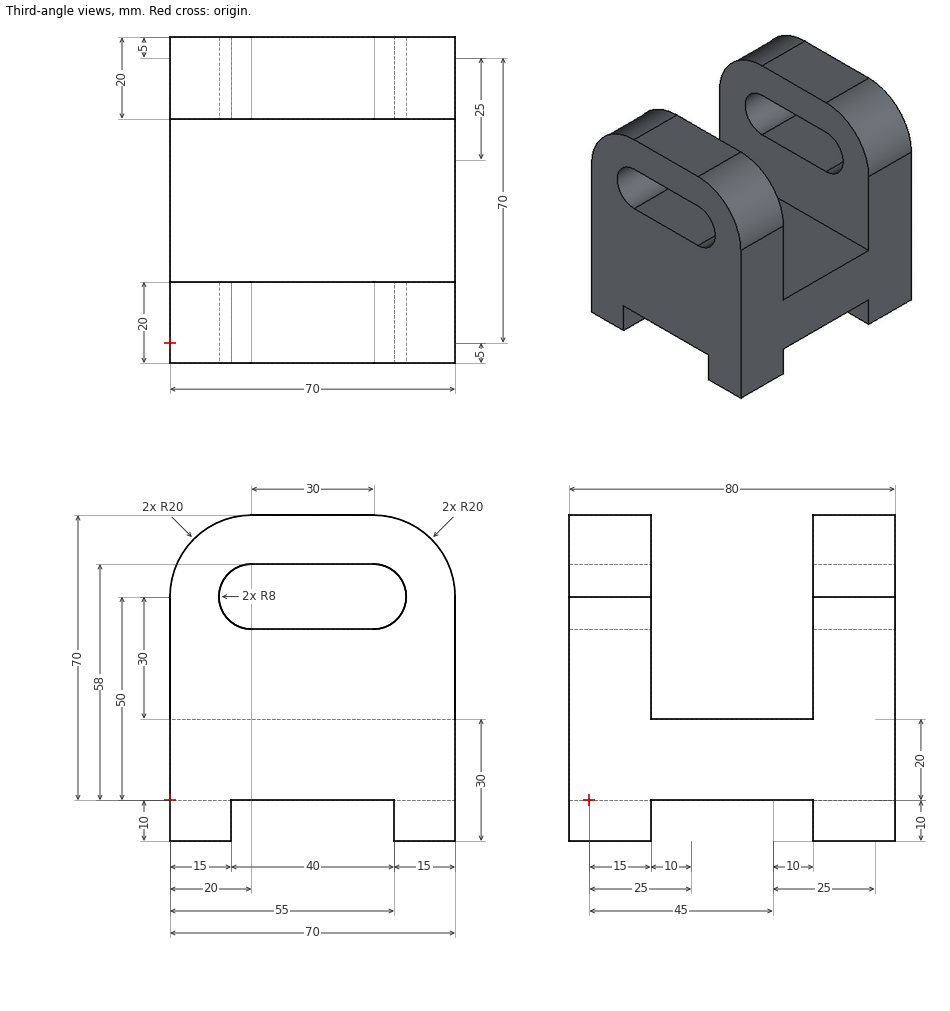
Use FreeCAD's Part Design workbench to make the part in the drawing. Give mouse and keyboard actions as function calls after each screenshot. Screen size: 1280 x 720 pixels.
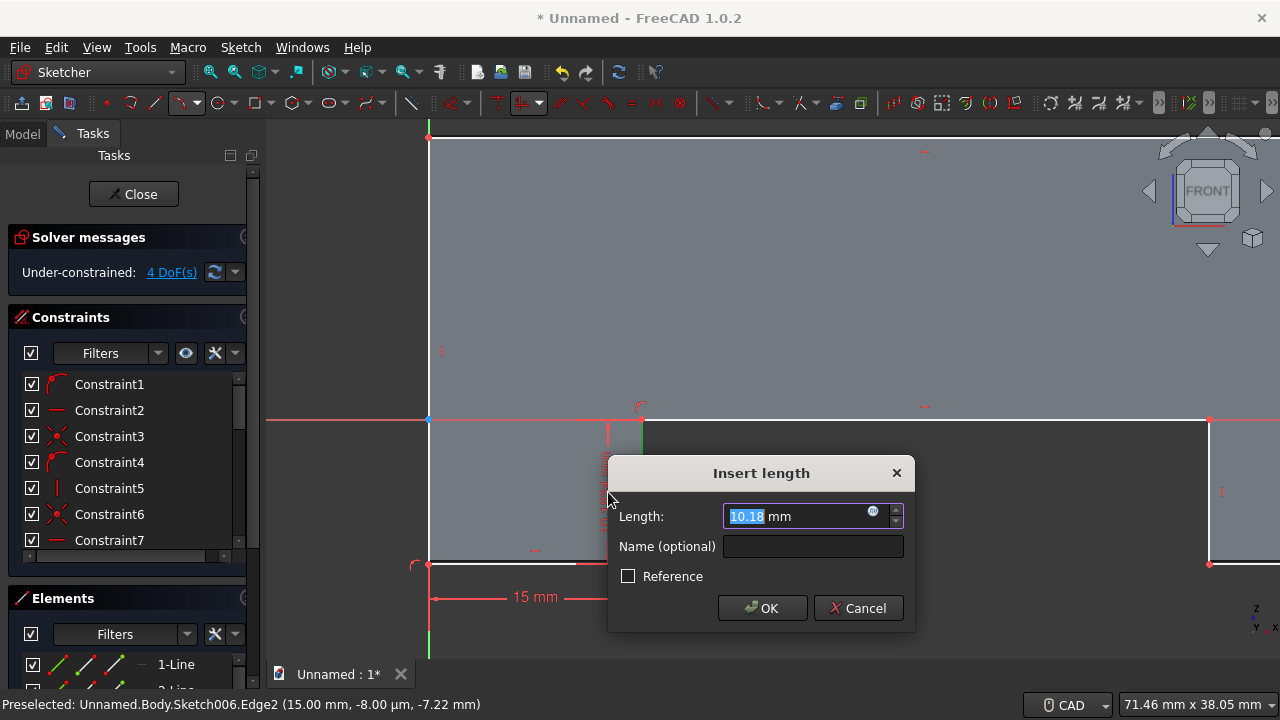
text(10)
key(Return)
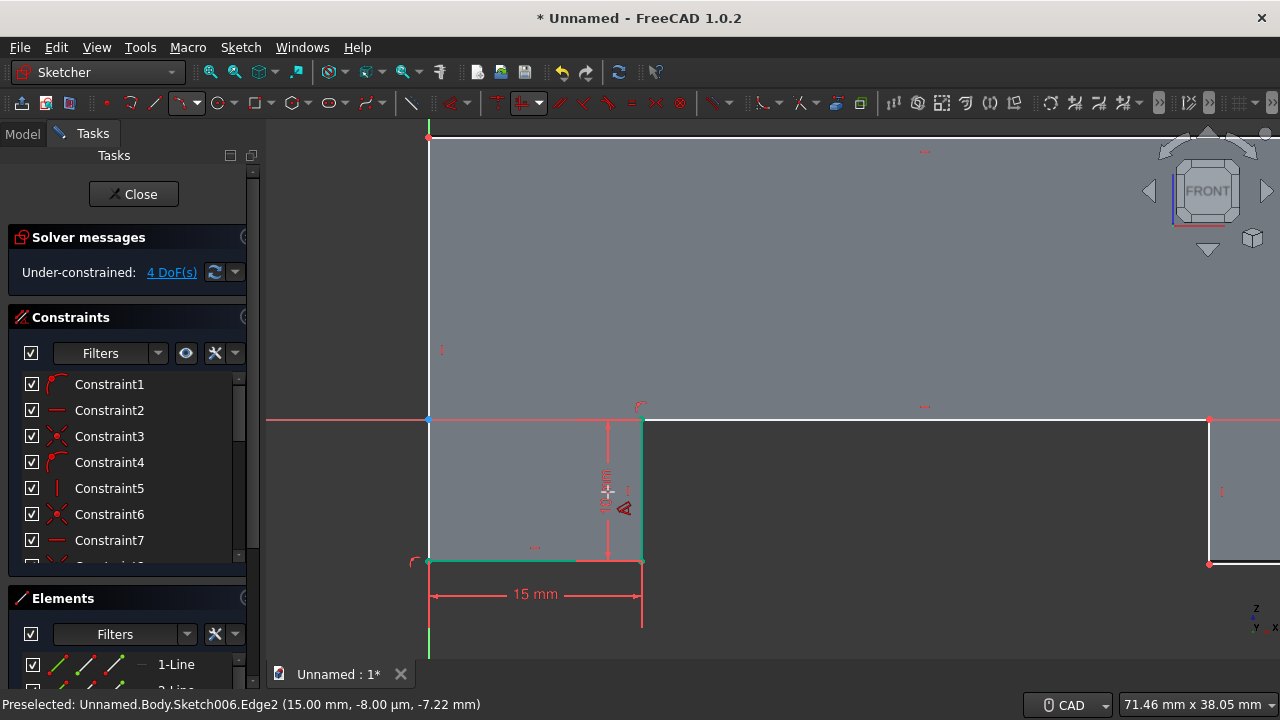
click(812, 420)
click(878, 454)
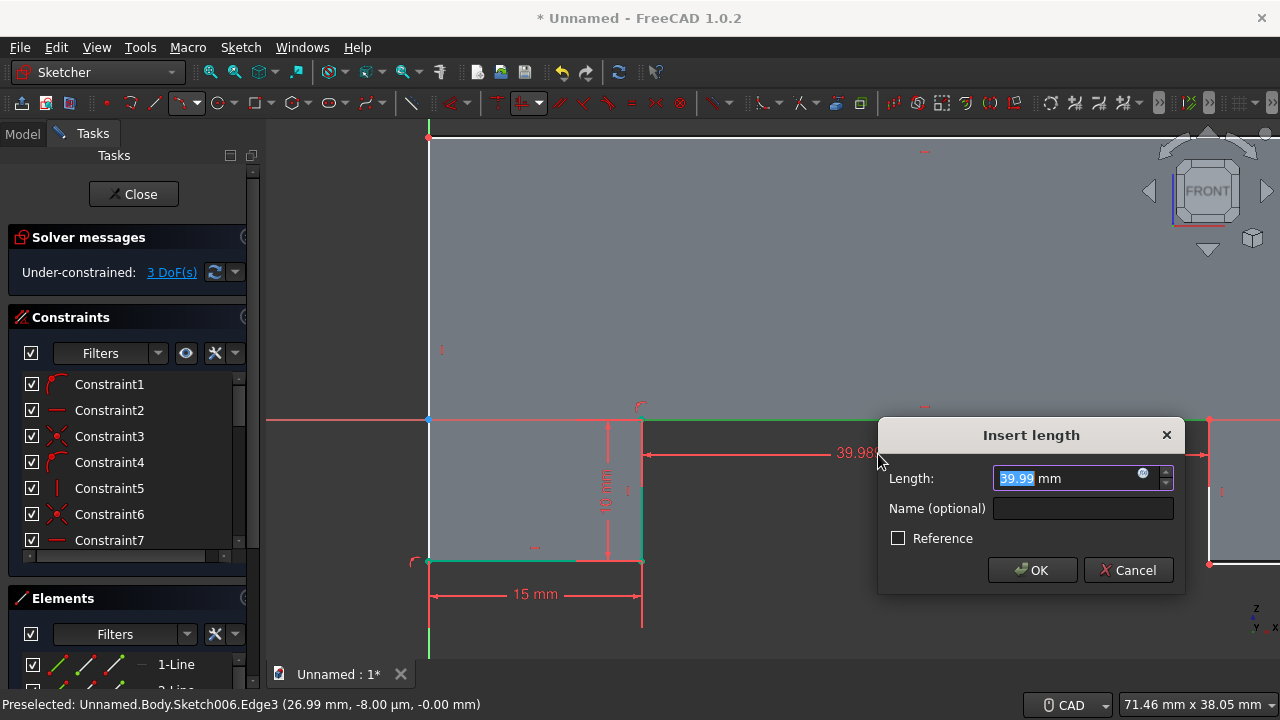
text(40)
key(Return)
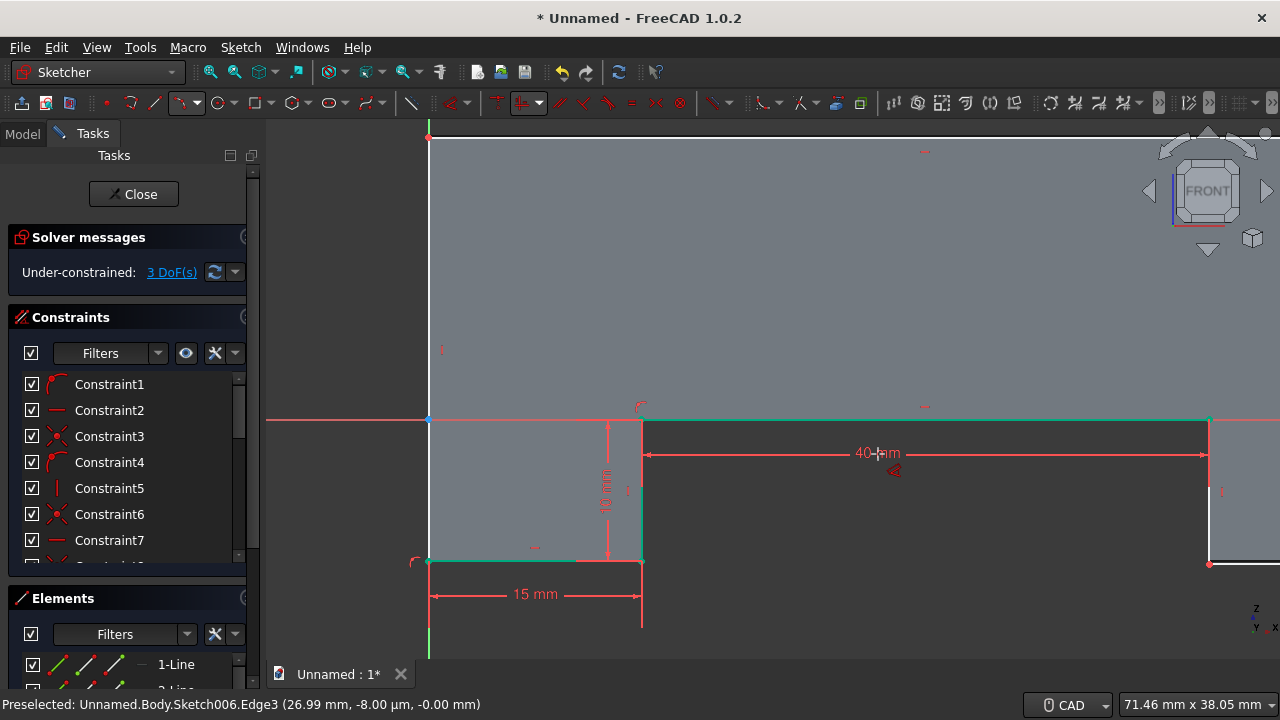
scroll(436, 438, down, 3)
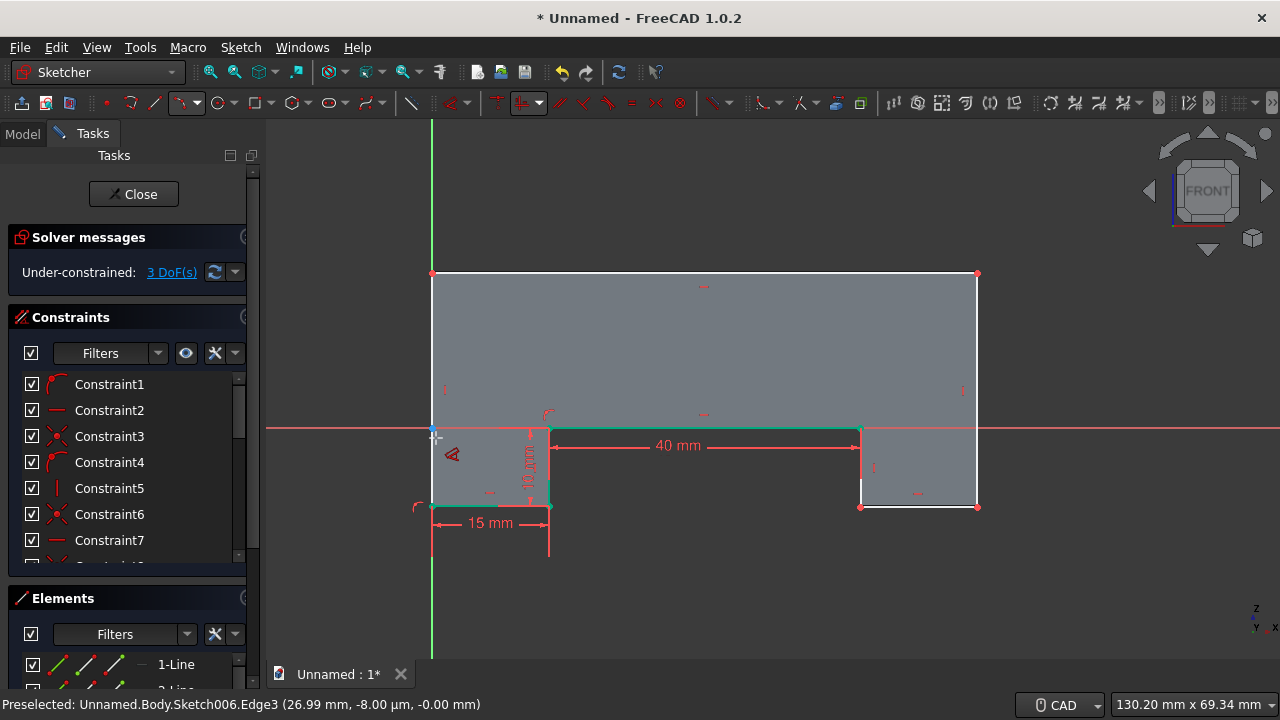
click(861, 452)
click(895, 468)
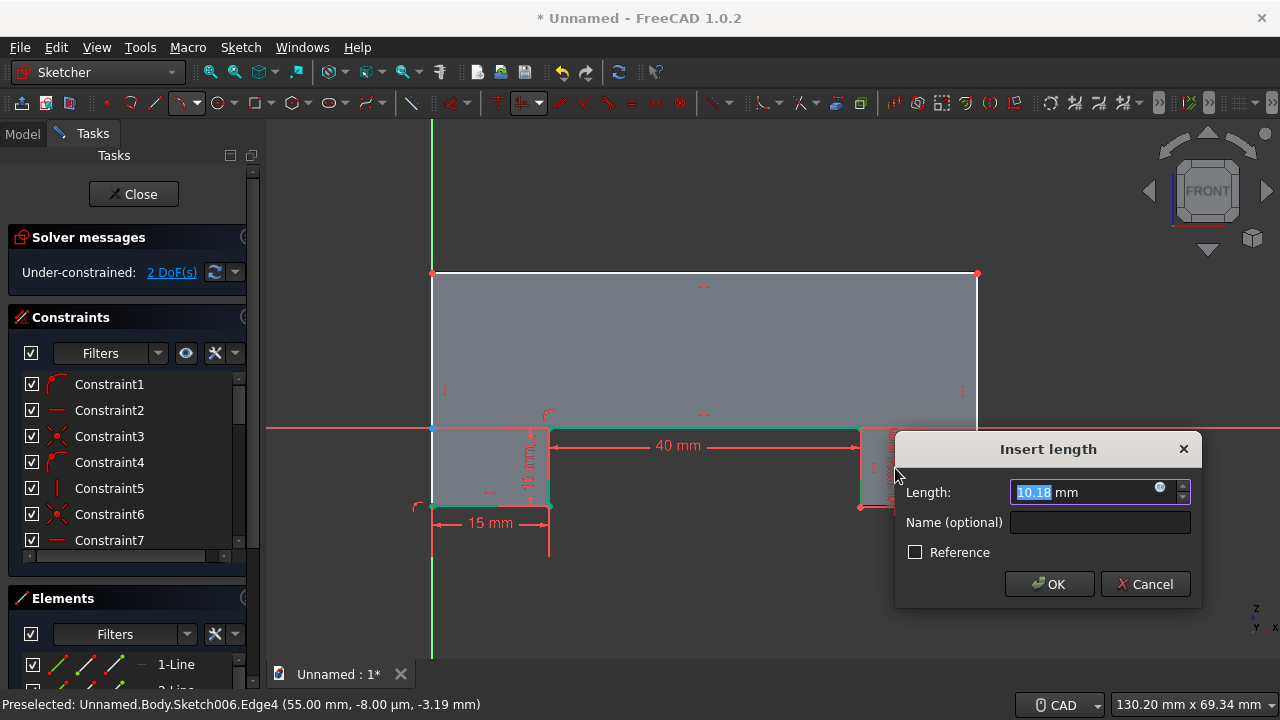
text(10)
key(Return)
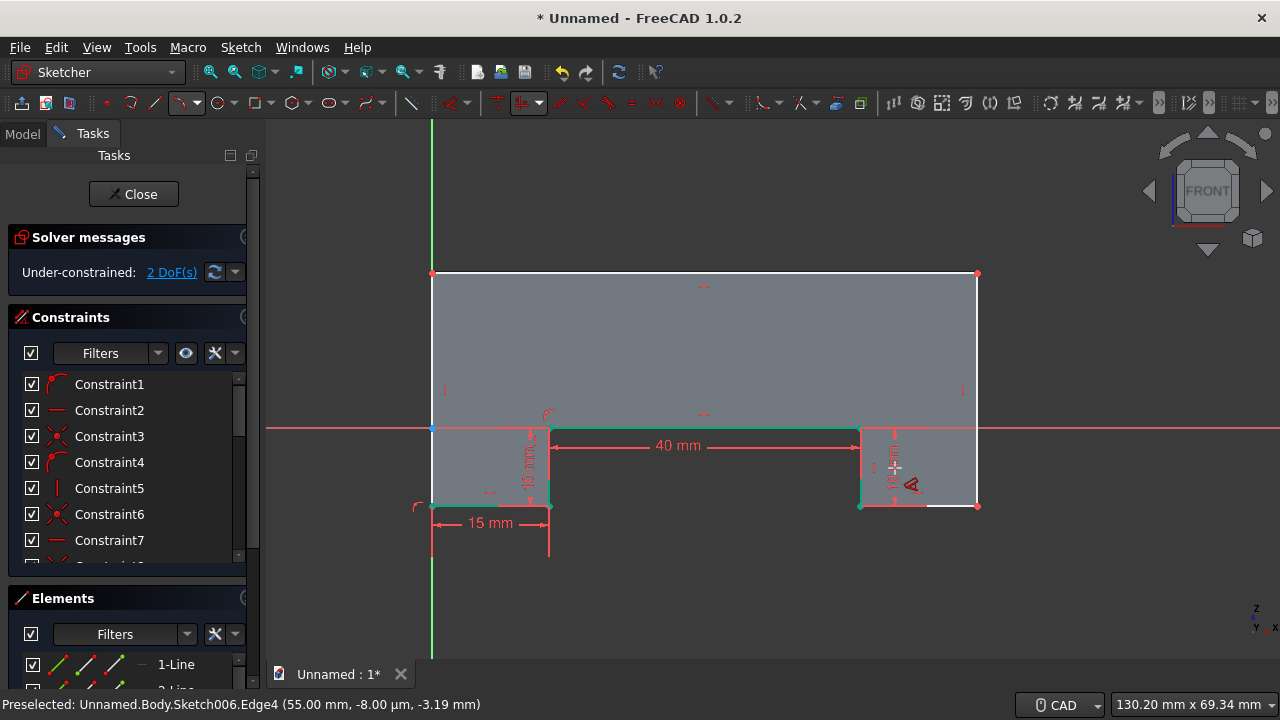
click(896, 506)
click(919, 540)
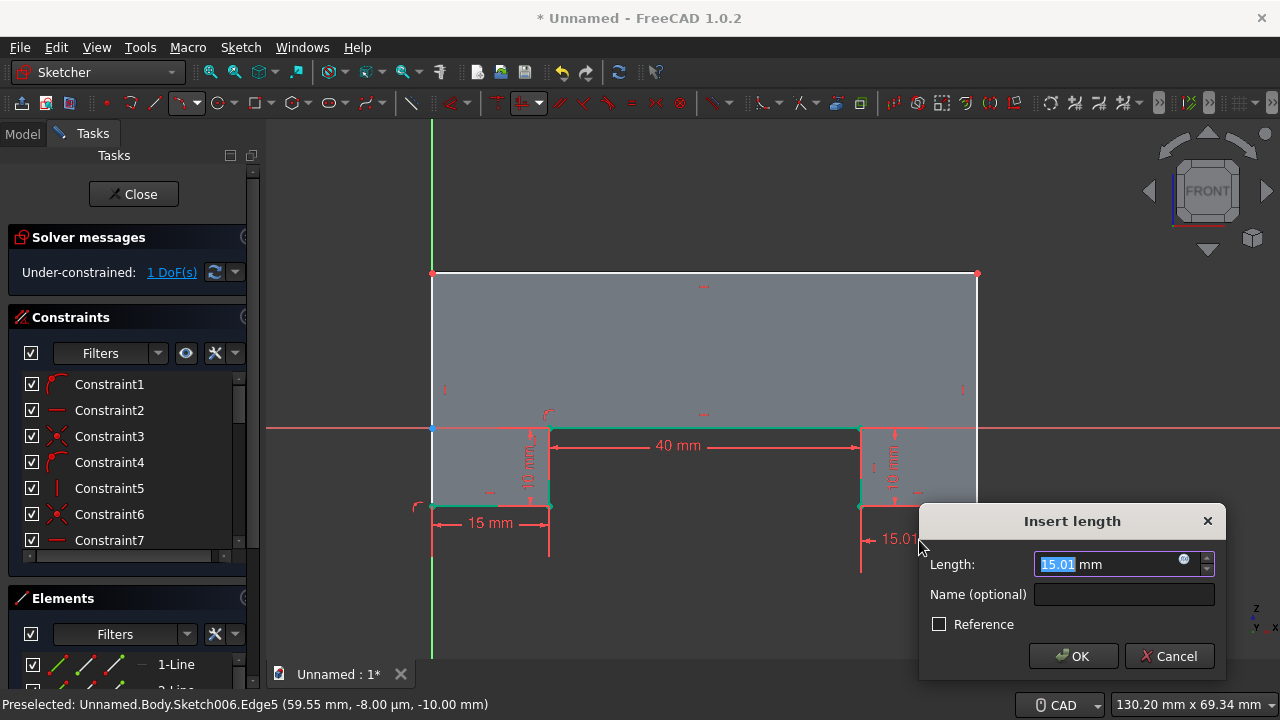
text(15)
key(Return)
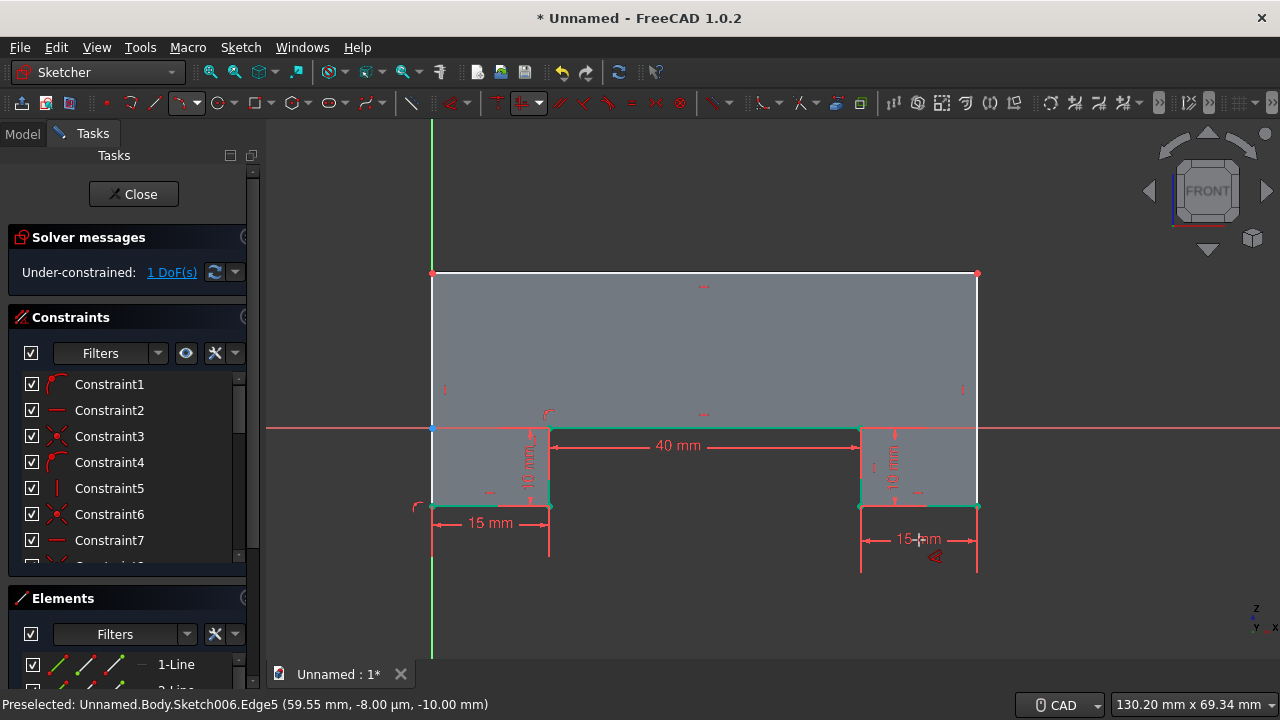
click(977, 343)
click(1011, 390)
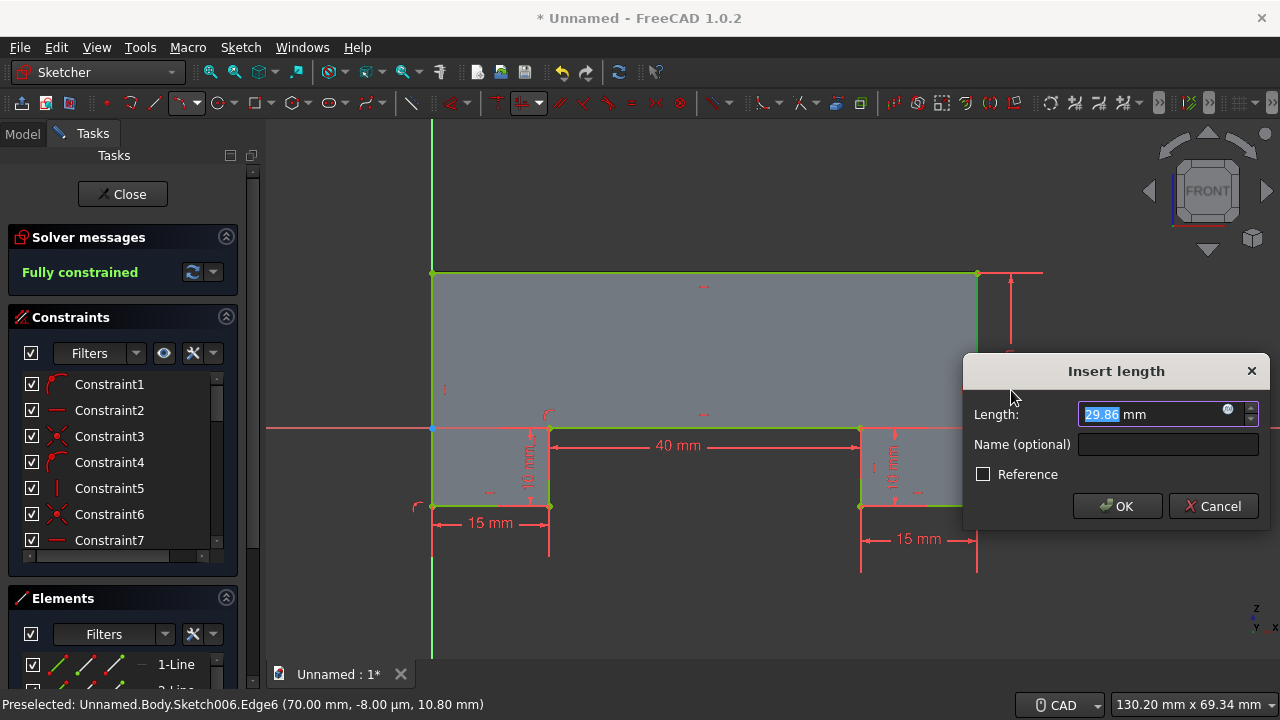
text(30)
key(Return)
key(Escape)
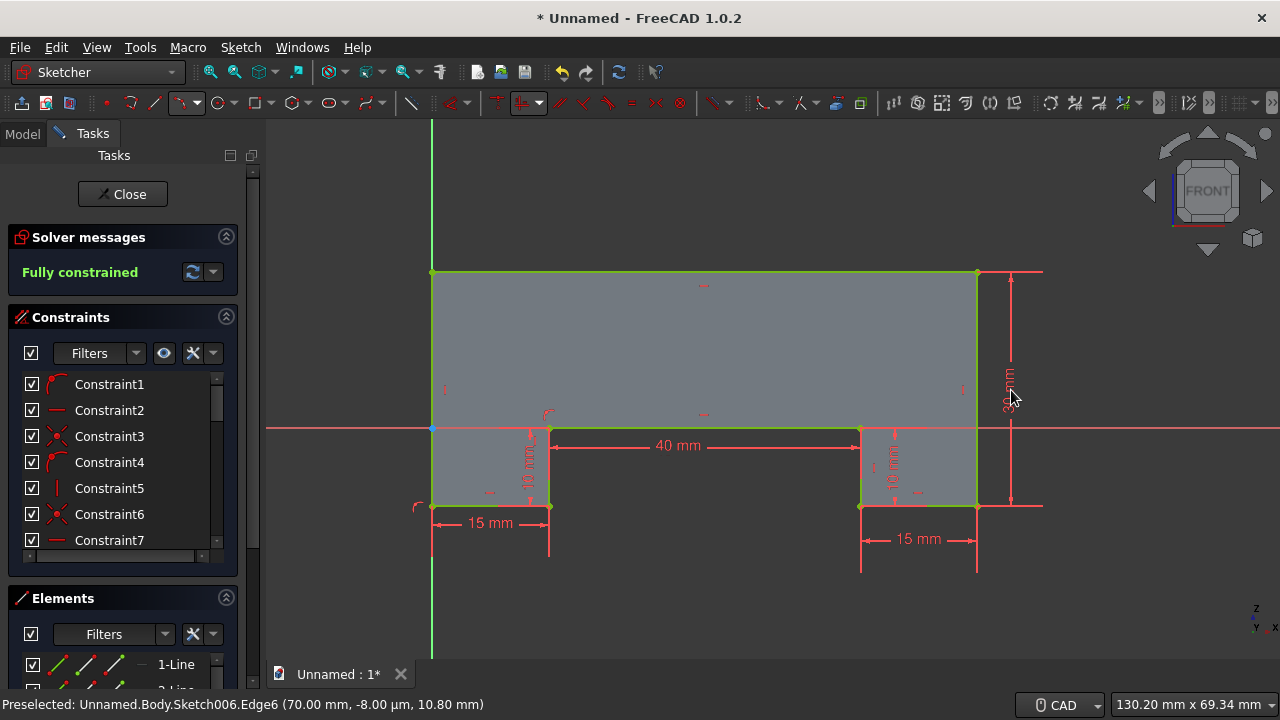
click(123, 194)